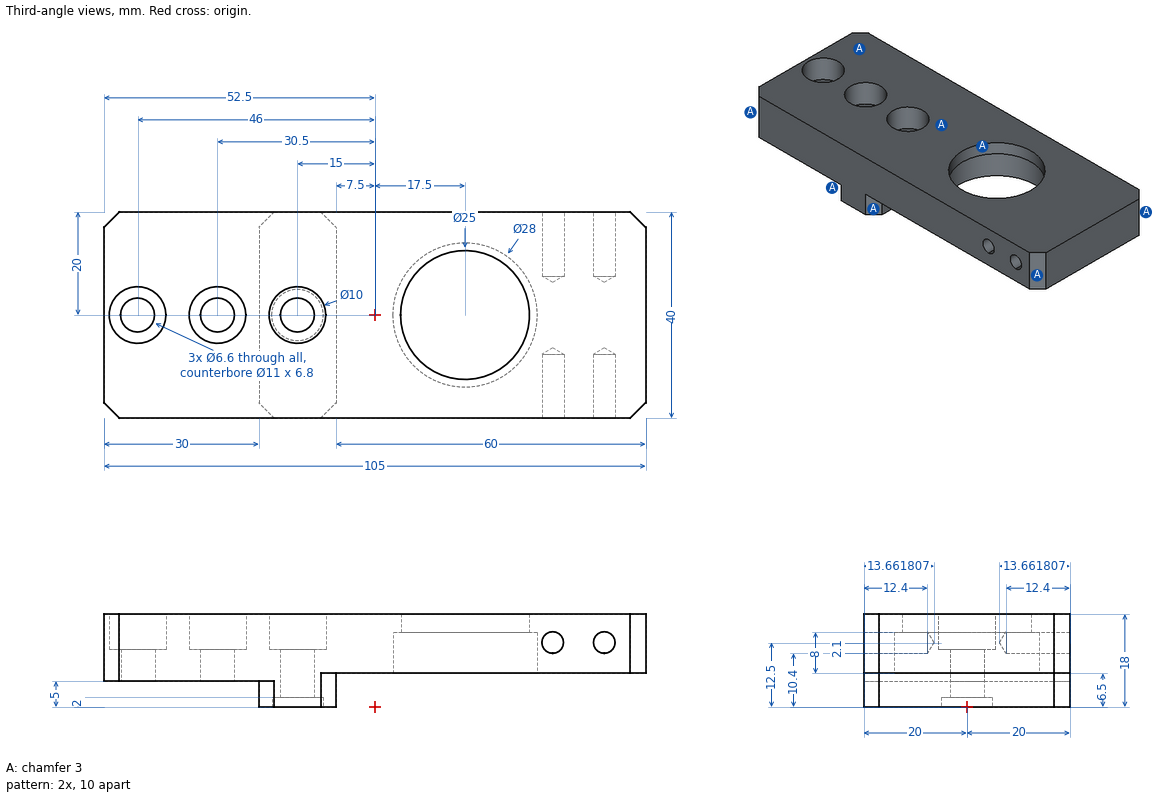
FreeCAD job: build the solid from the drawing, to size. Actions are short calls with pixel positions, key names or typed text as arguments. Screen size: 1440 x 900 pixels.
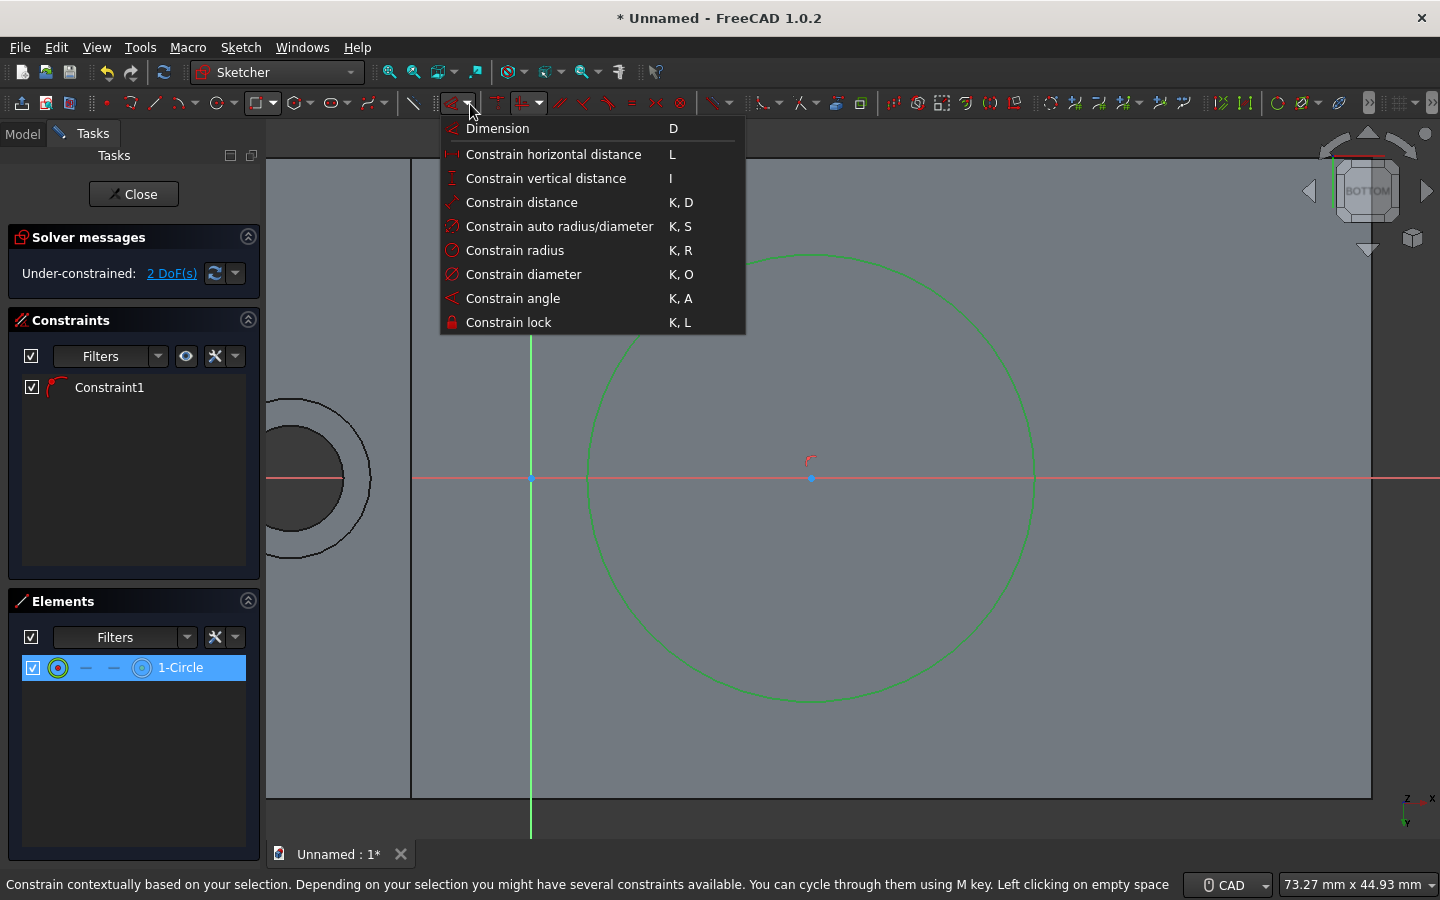
click(593, 274)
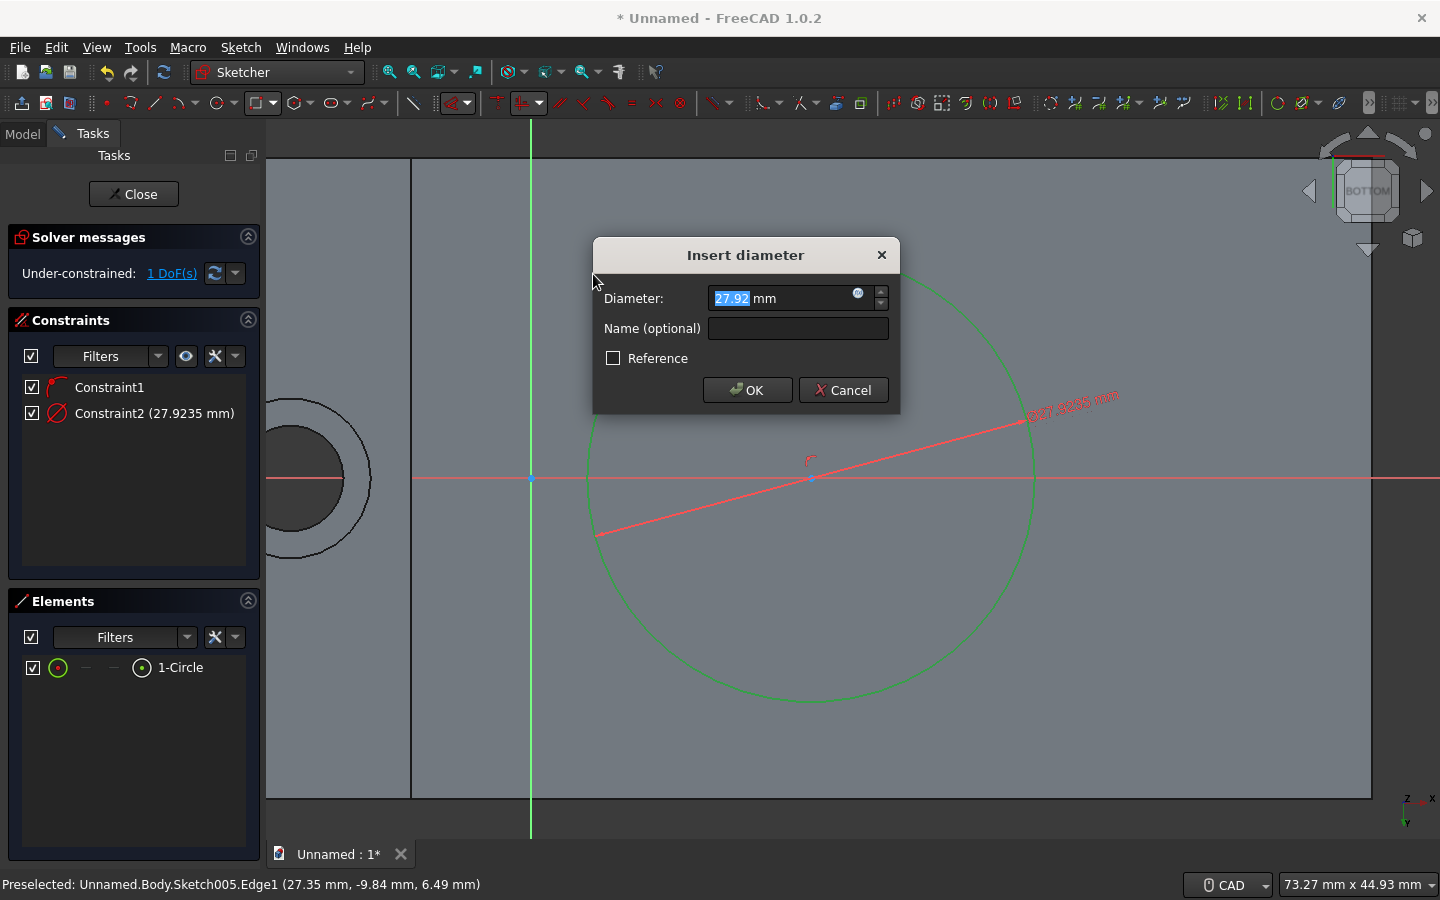
text(28)
key(Return)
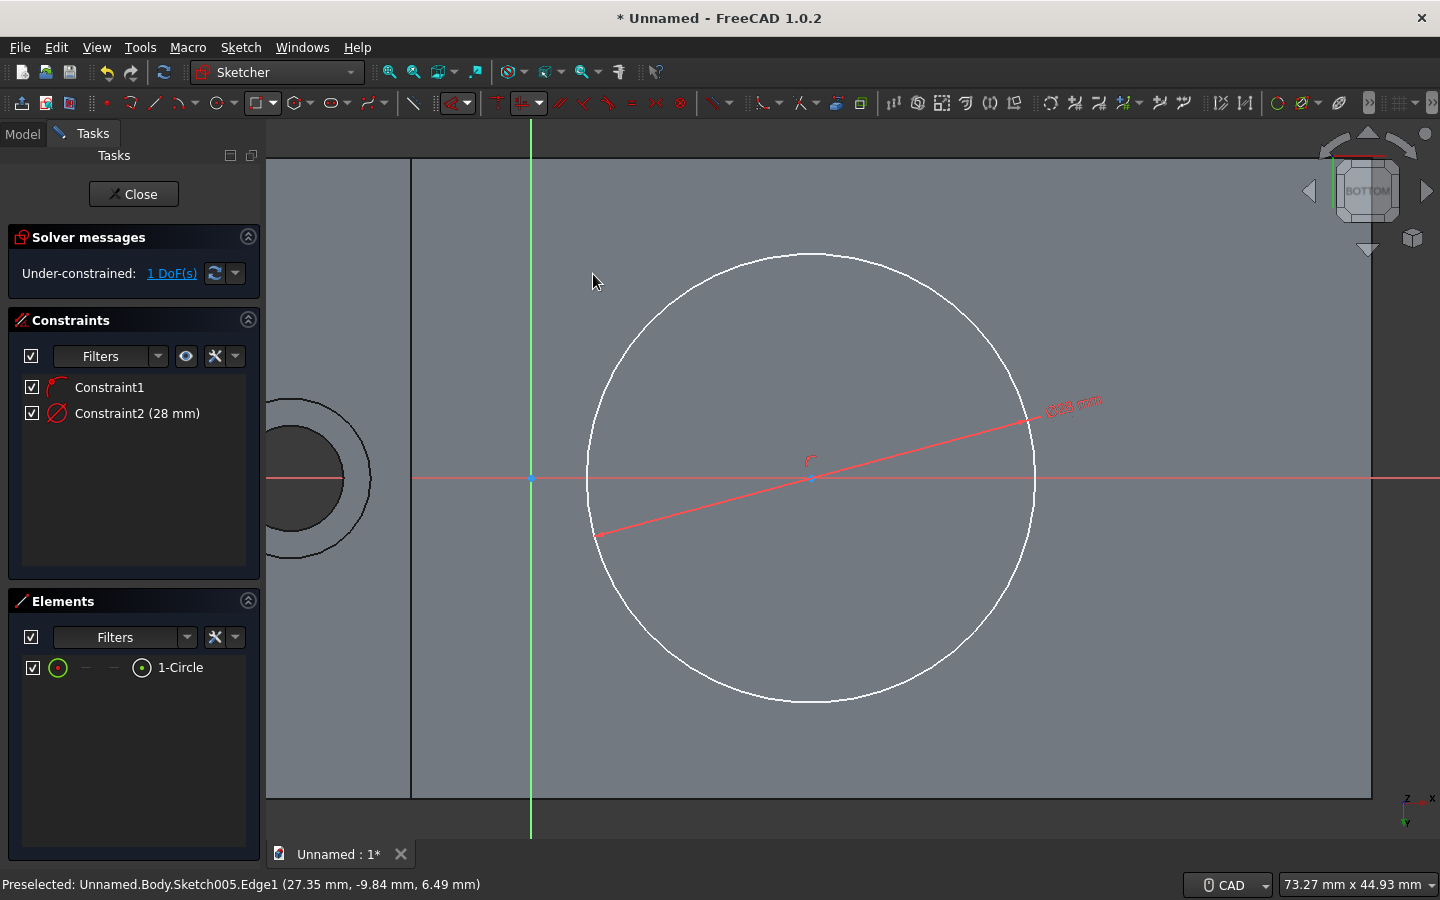
click(811, 478)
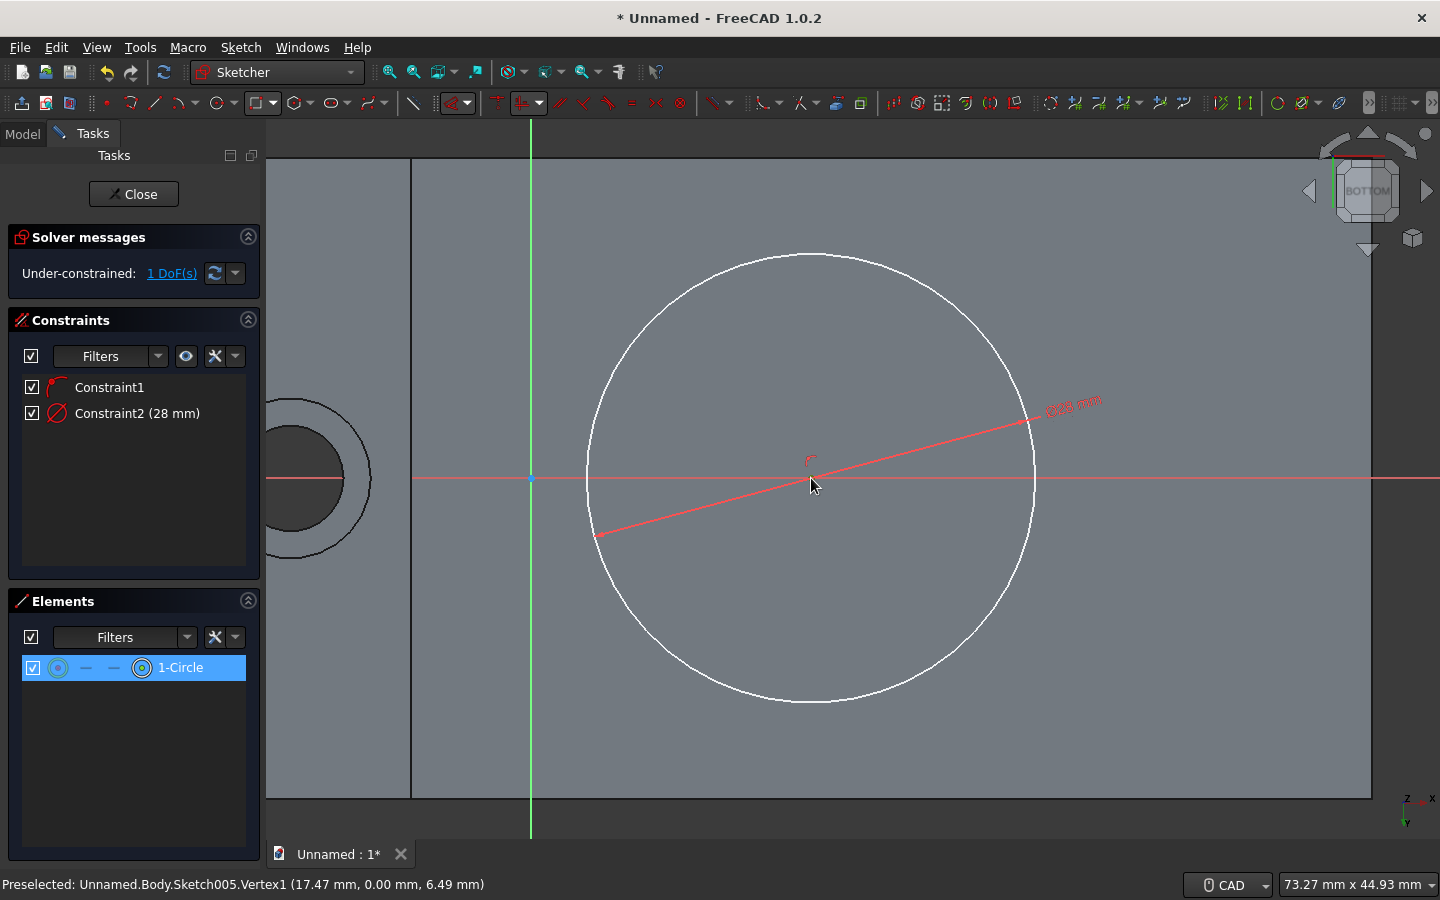
key(l)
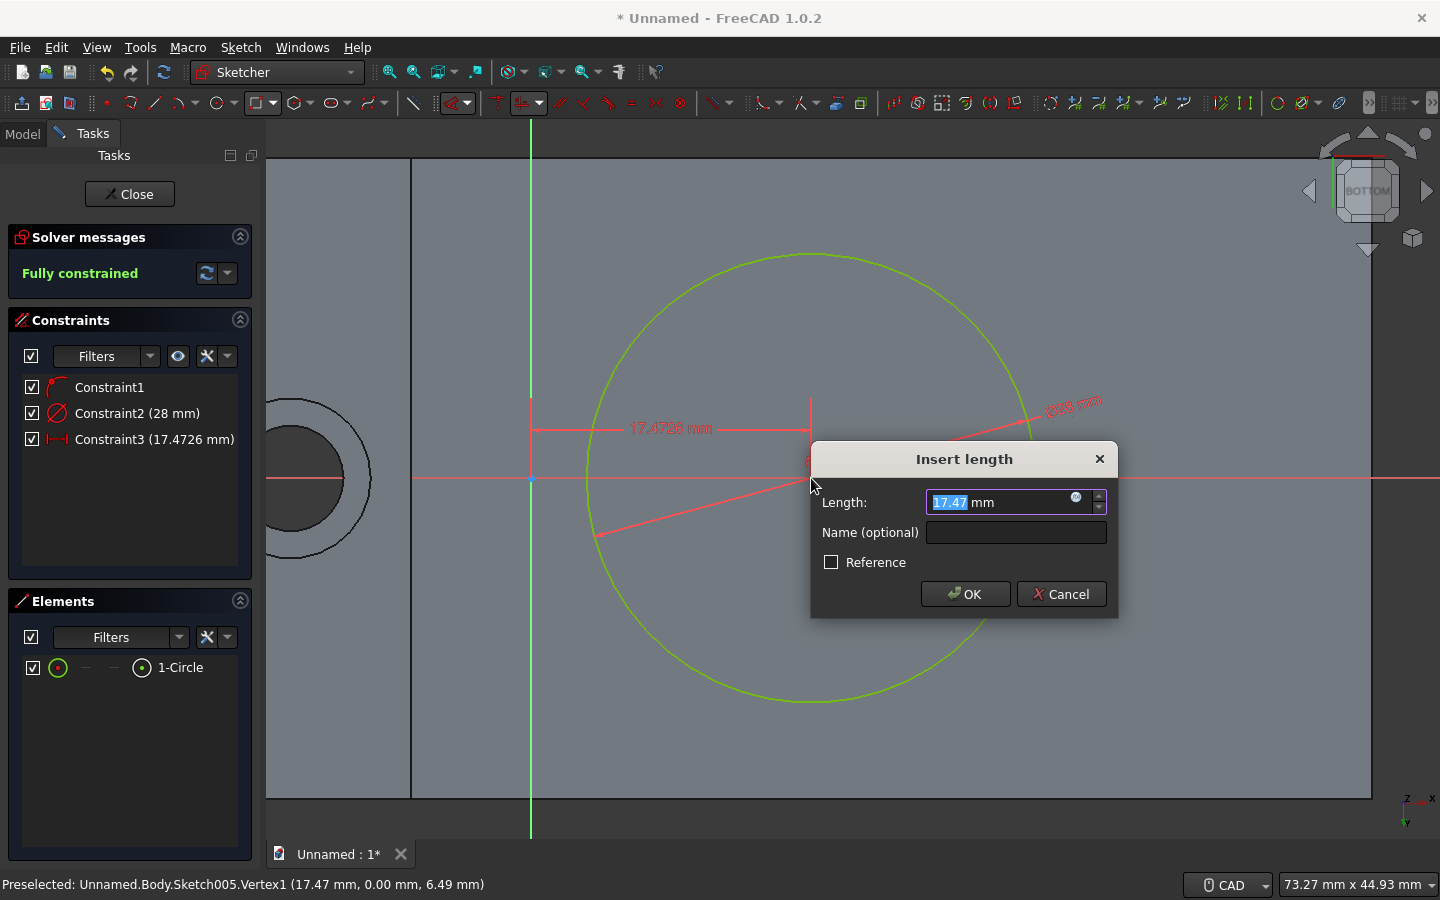
text(17.5)
key(Return)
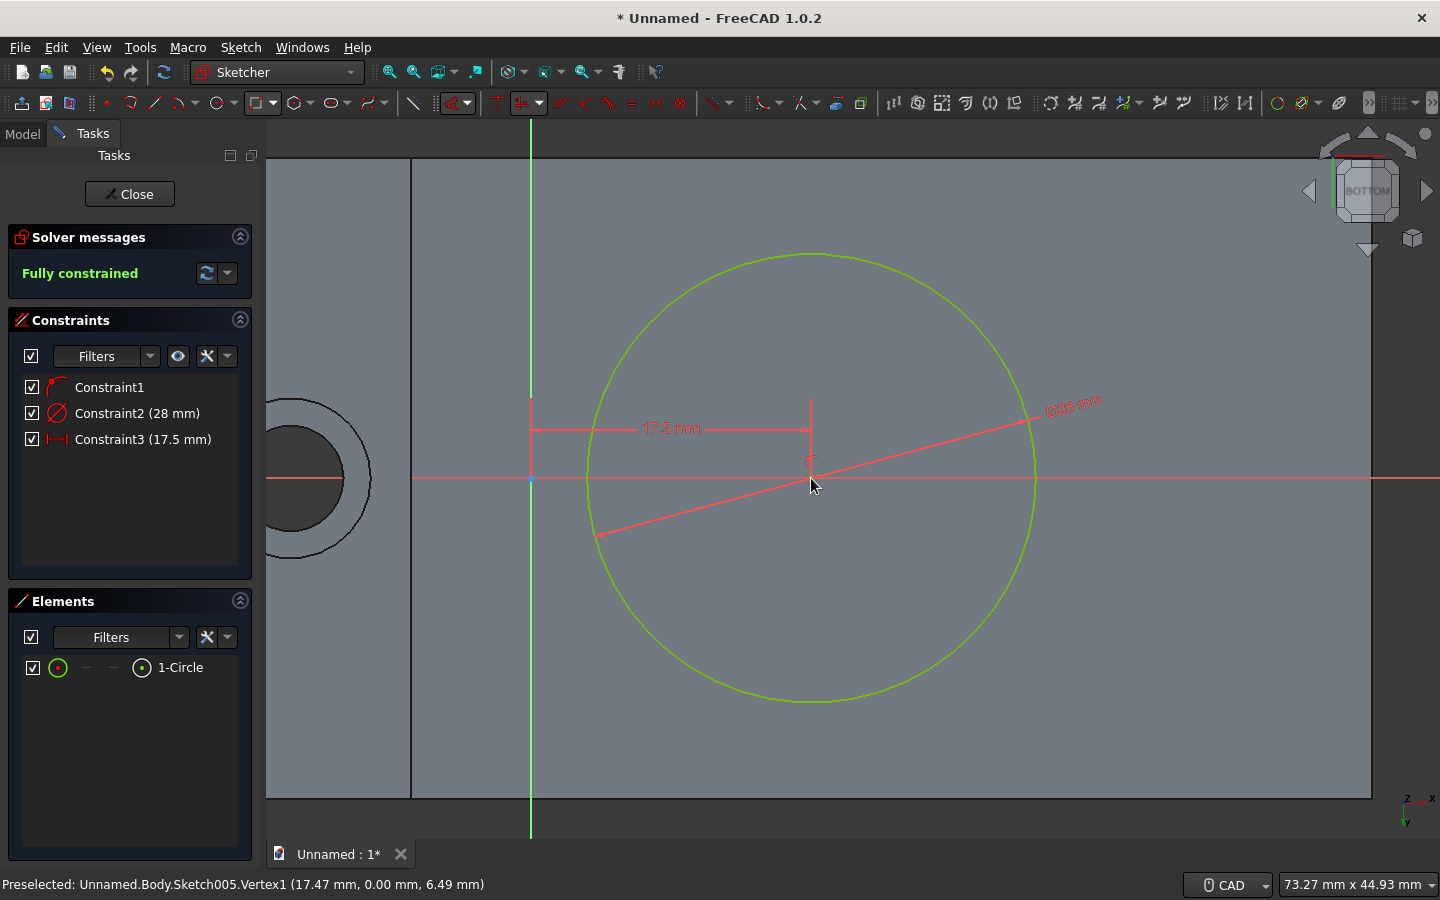
click(130, 194)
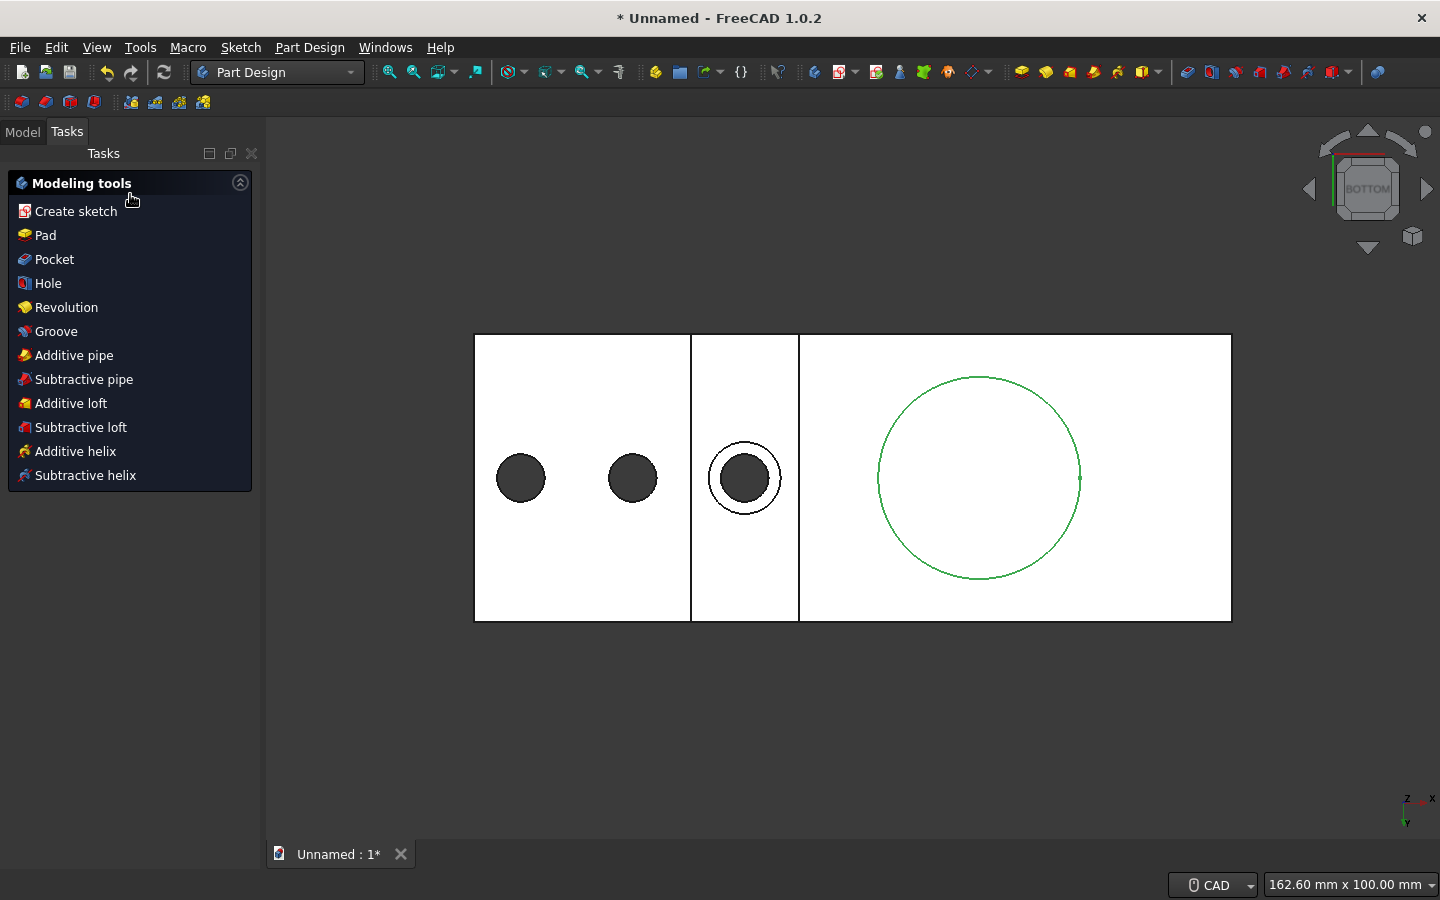
click(1188, 72)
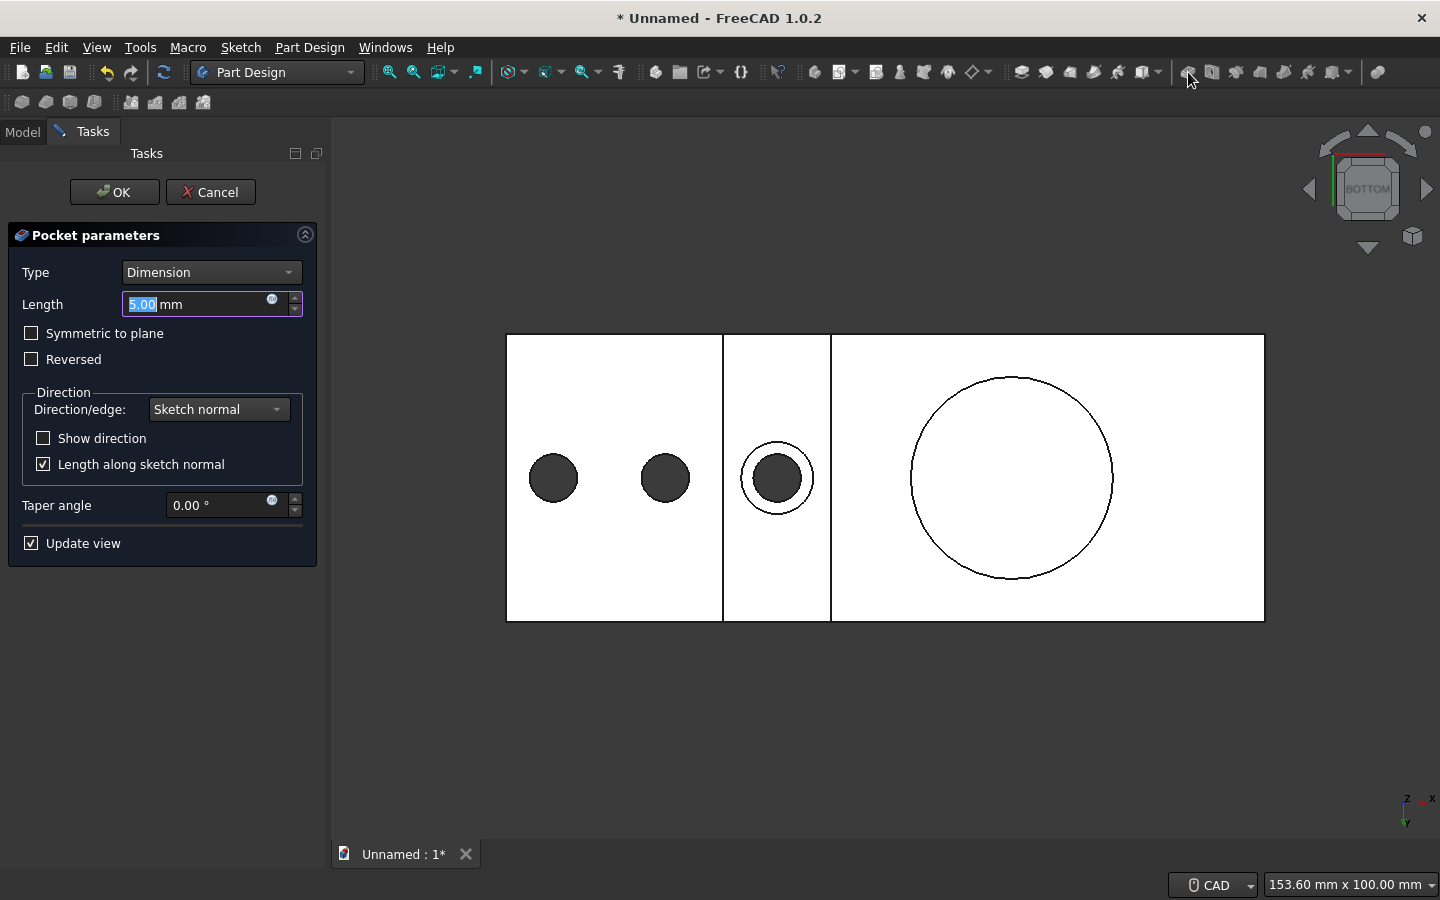
text(8)
key(Tab)